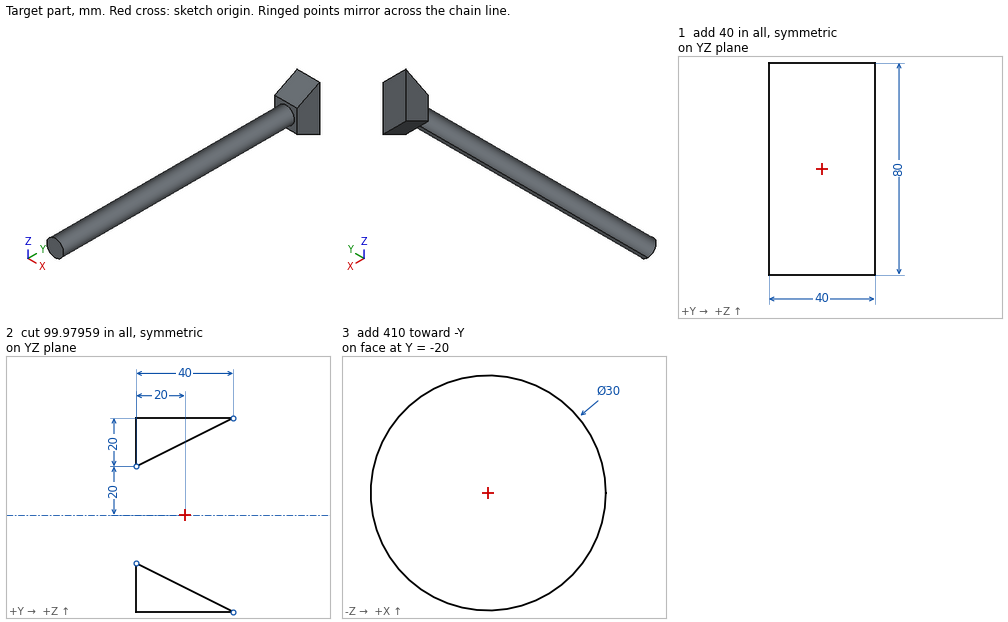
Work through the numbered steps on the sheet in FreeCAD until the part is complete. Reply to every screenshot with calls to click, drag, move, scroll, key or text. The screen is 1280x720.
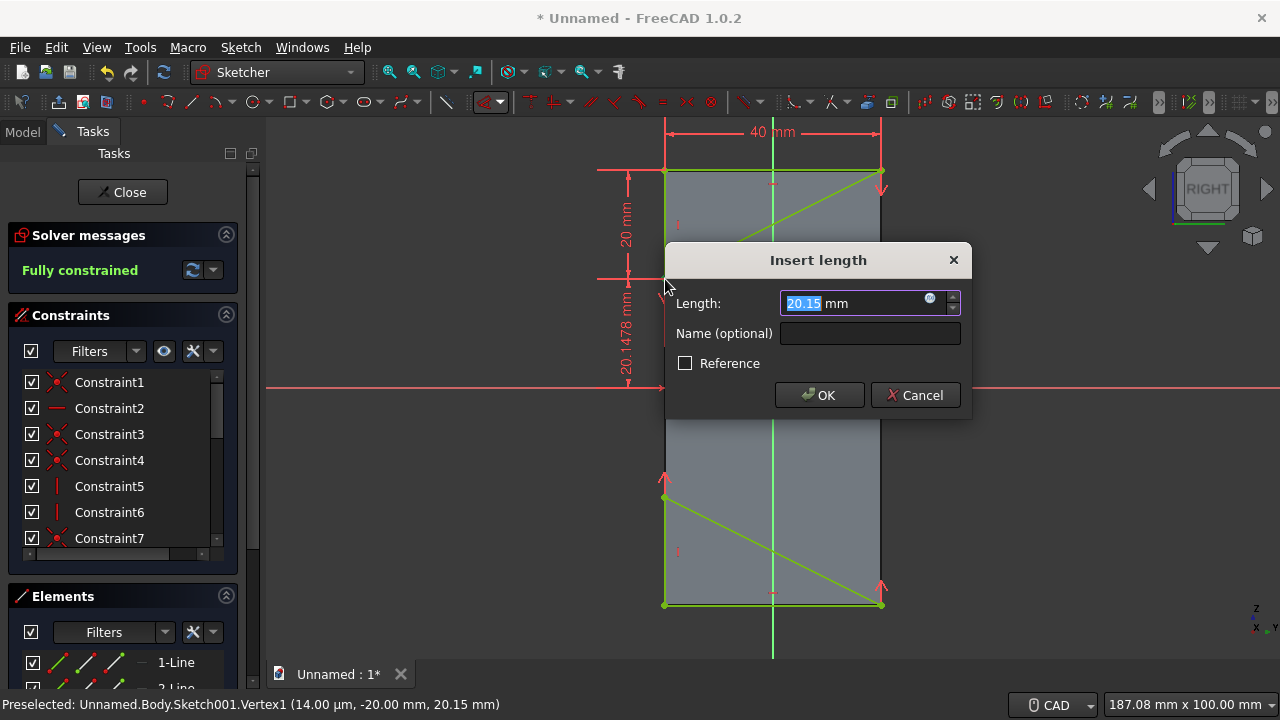
text(20)
key(Return)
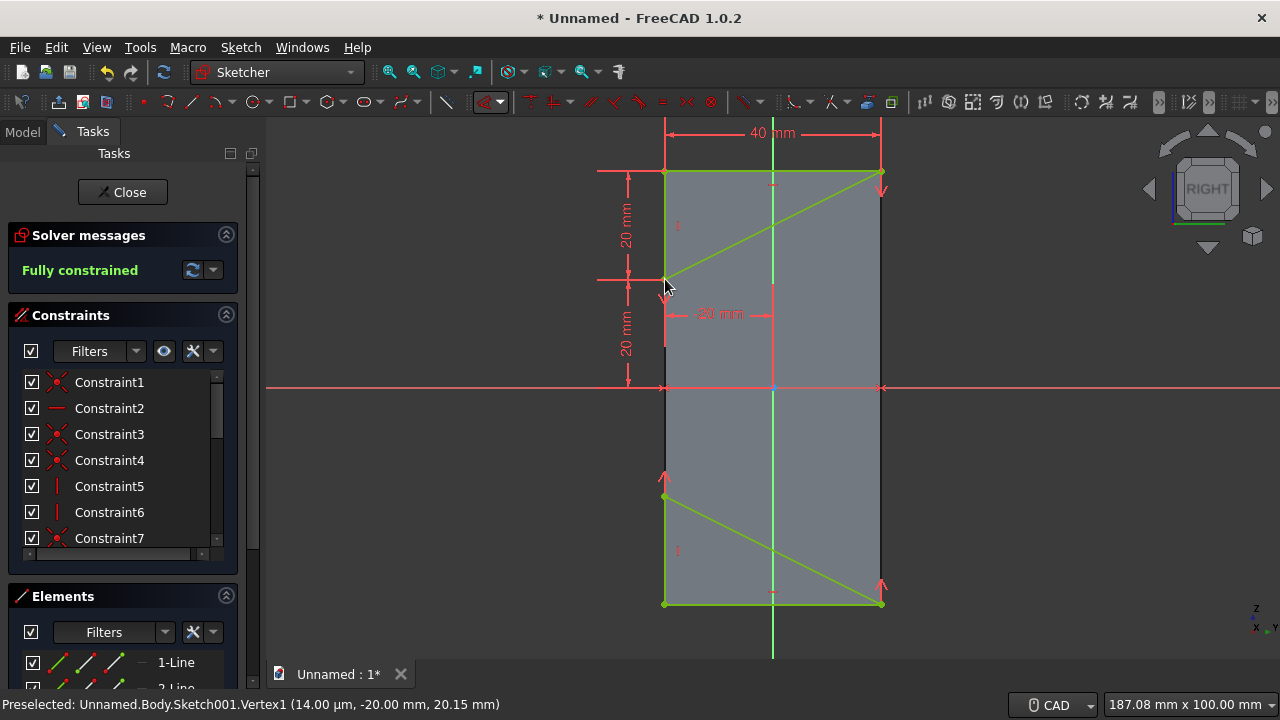
click(123, 192)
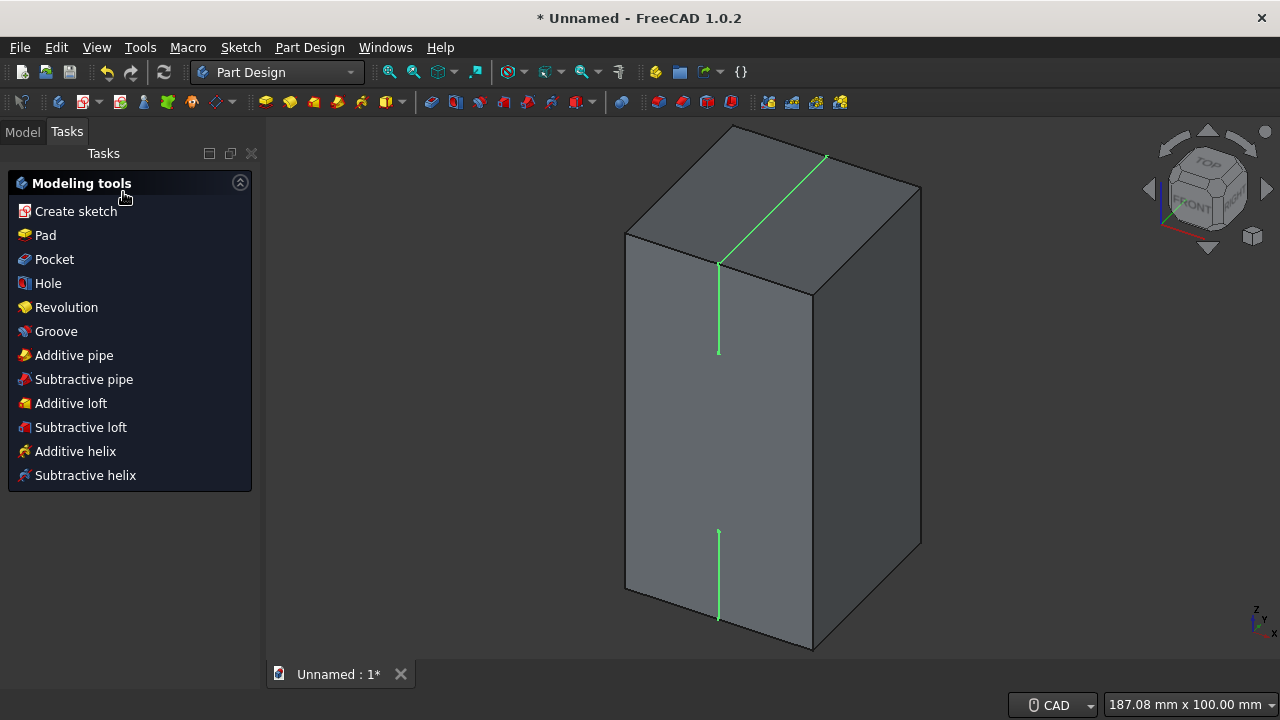
click(432, 102)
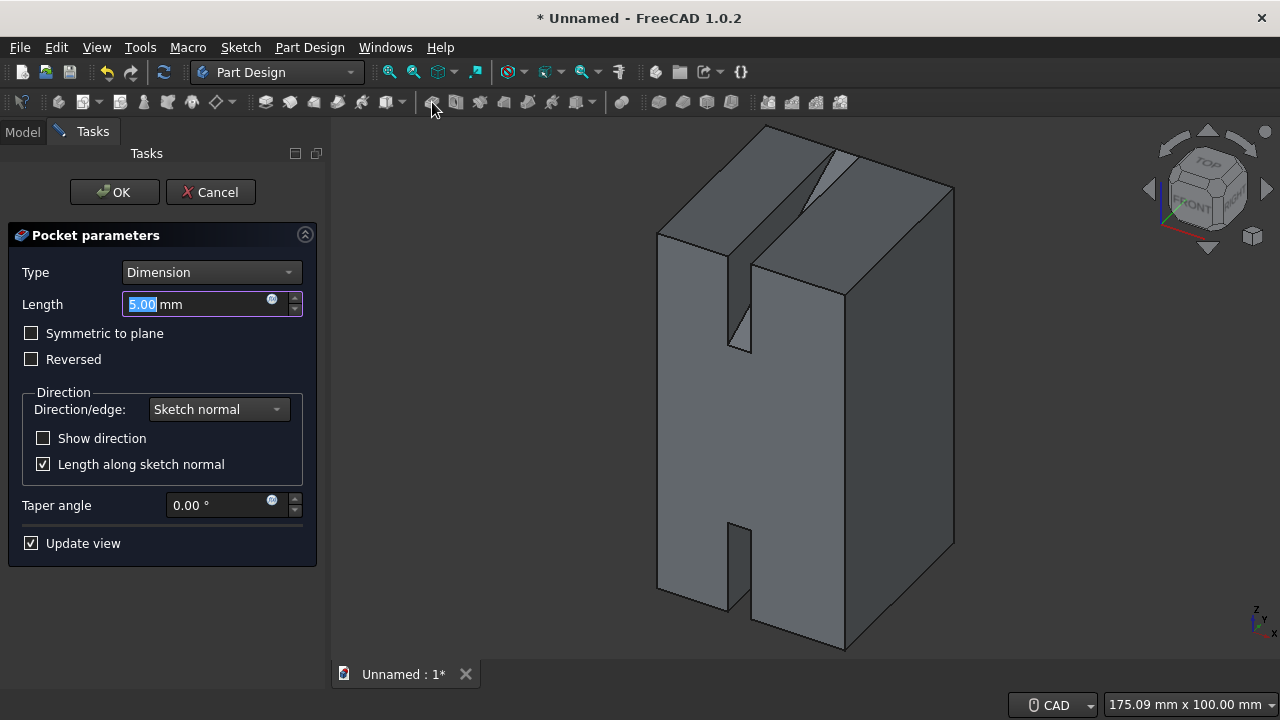
text(99.97959)
key(Tab)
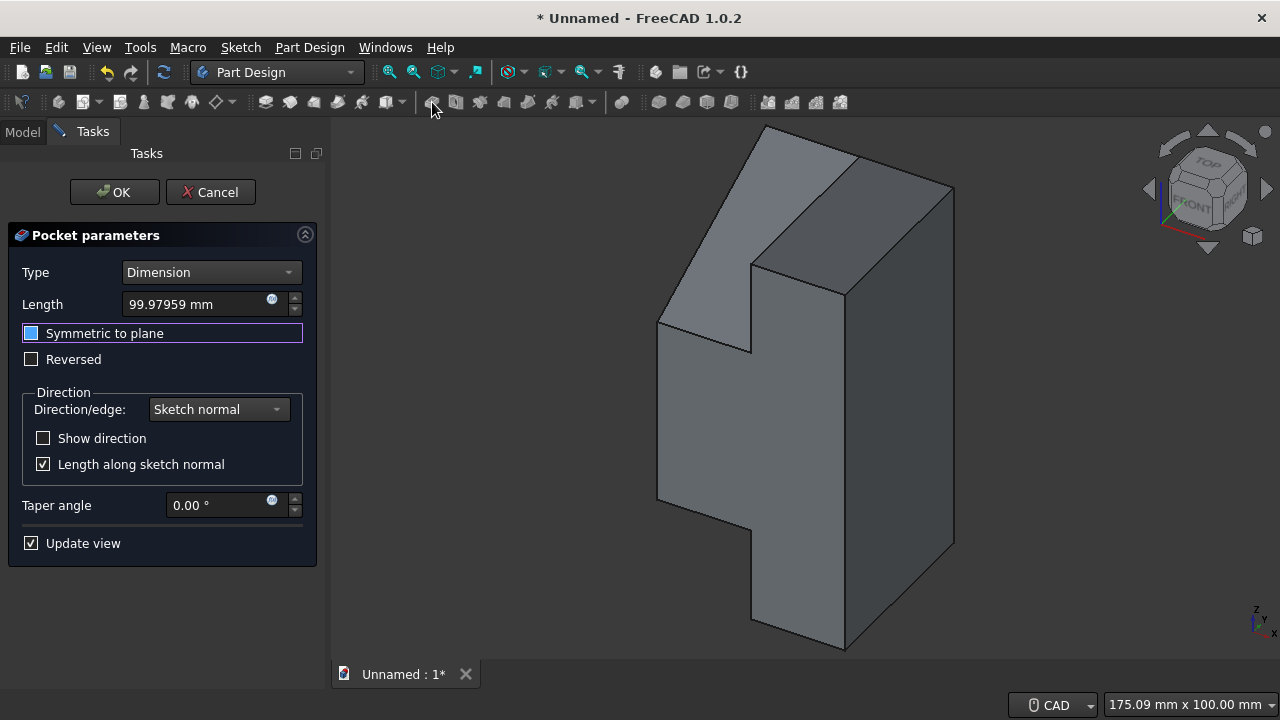
click(30, 333)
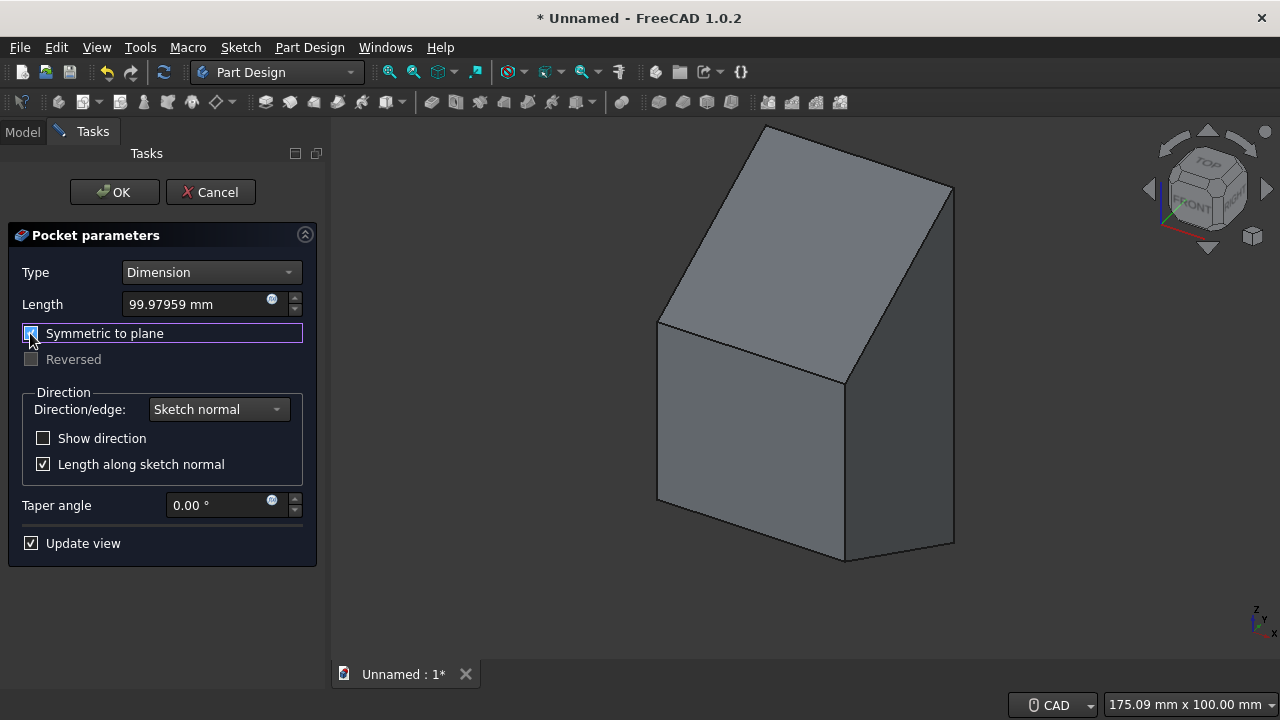
click(115, 192)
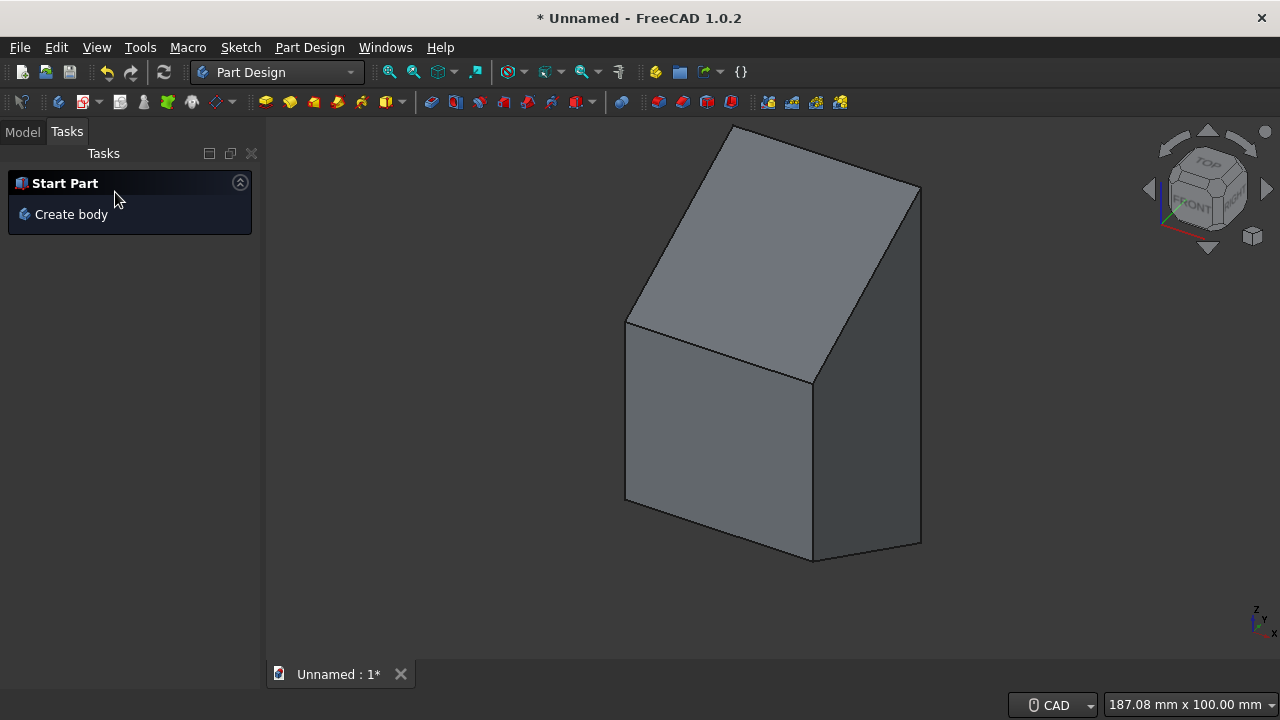
click(719, 441)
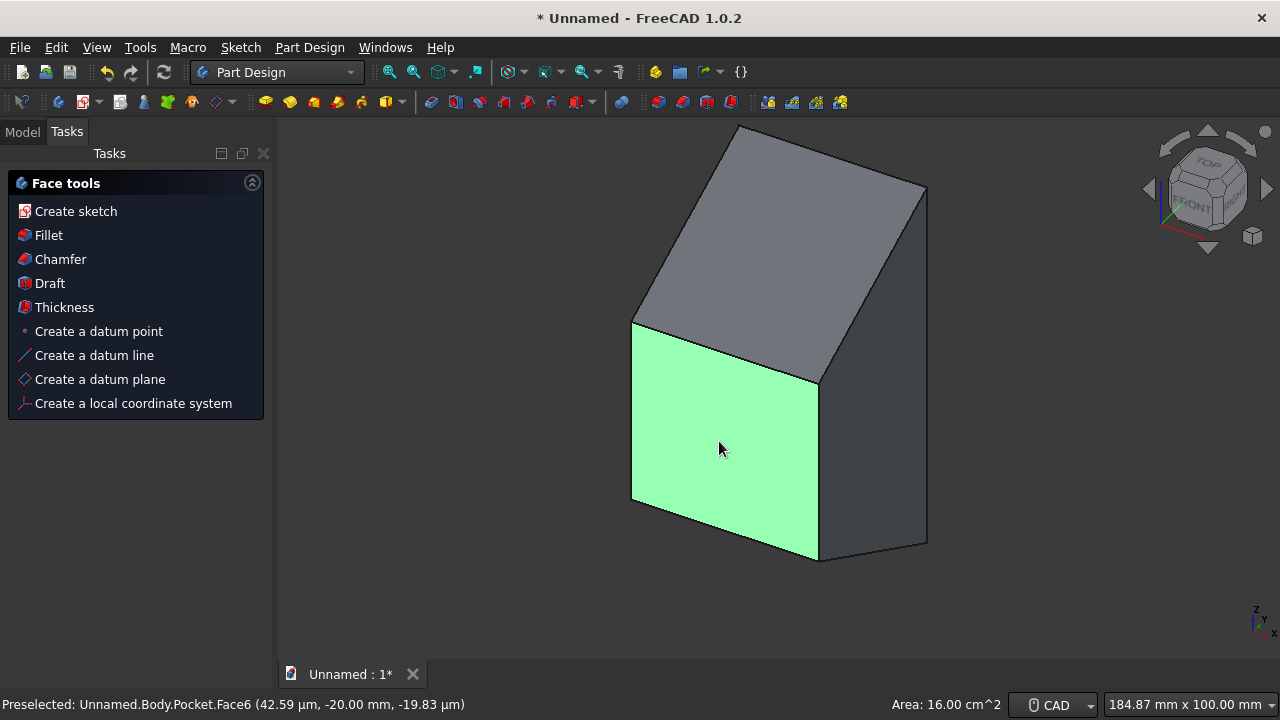
click(84, 102)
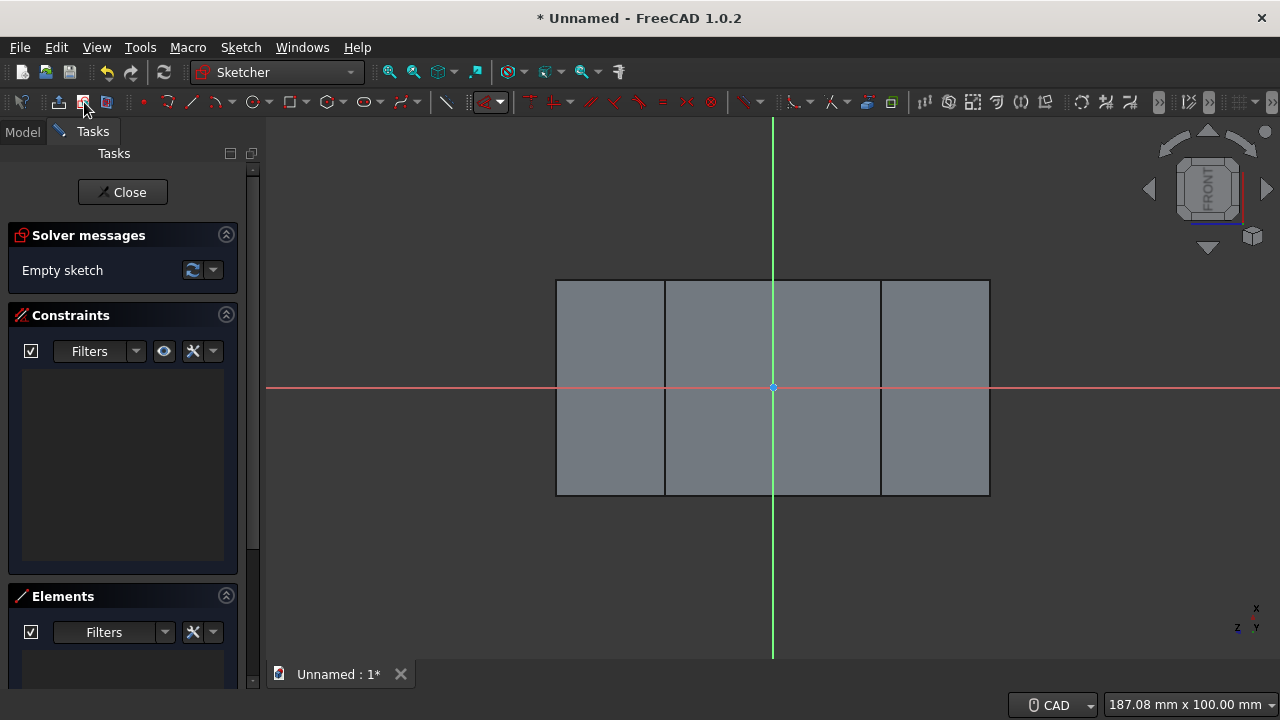
scroll(829, 388, up, 4)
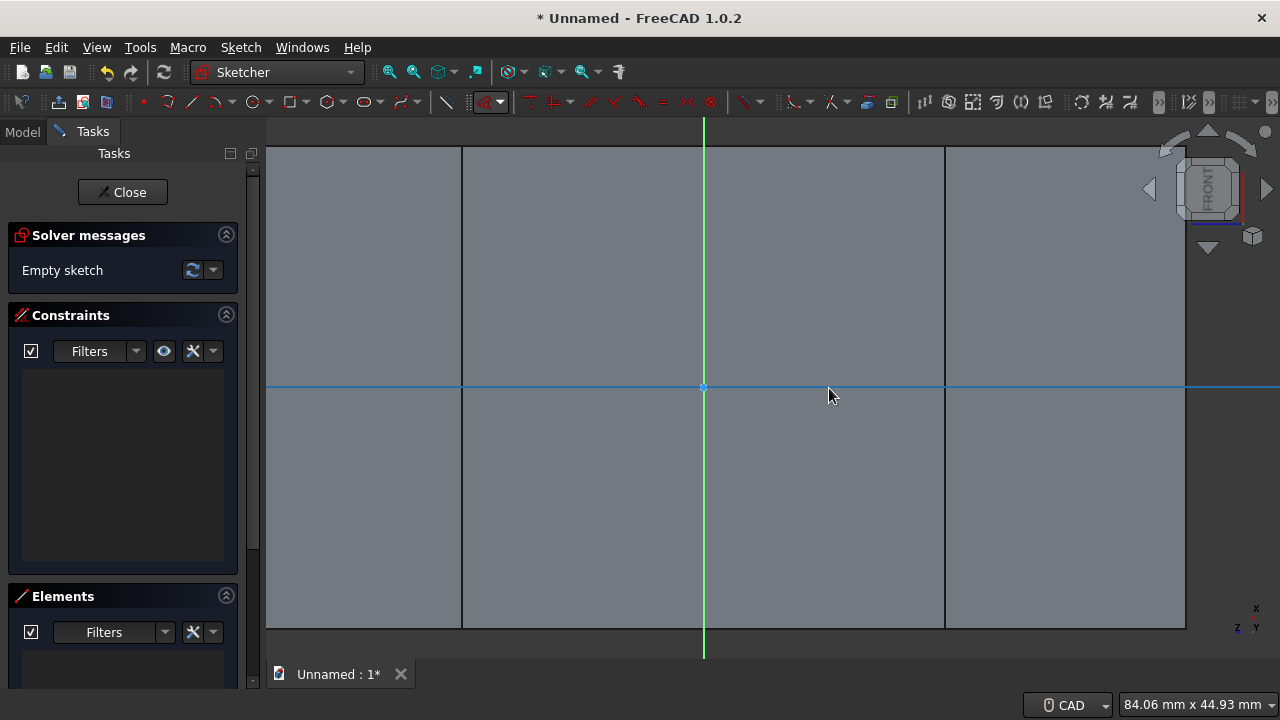
key(g)
key(c)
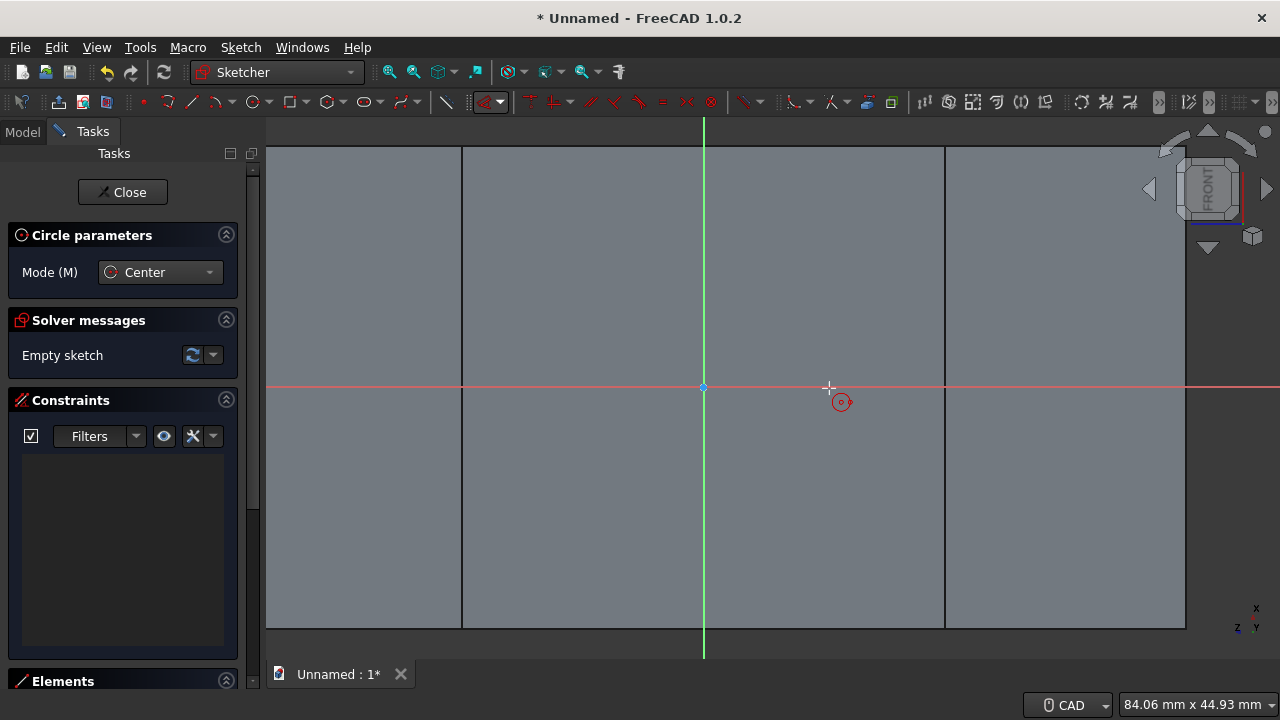
click(704, 387)
click(832, 259)
key(Escape)